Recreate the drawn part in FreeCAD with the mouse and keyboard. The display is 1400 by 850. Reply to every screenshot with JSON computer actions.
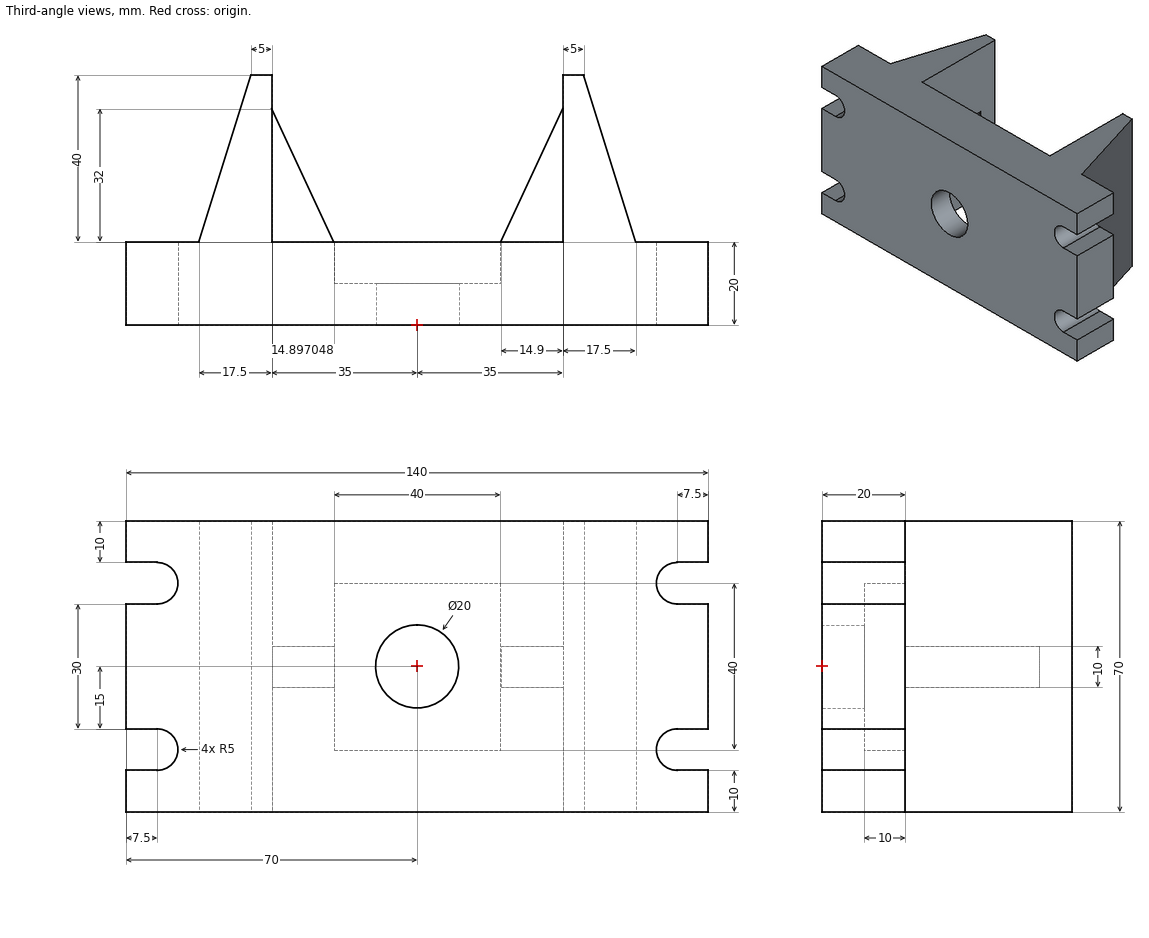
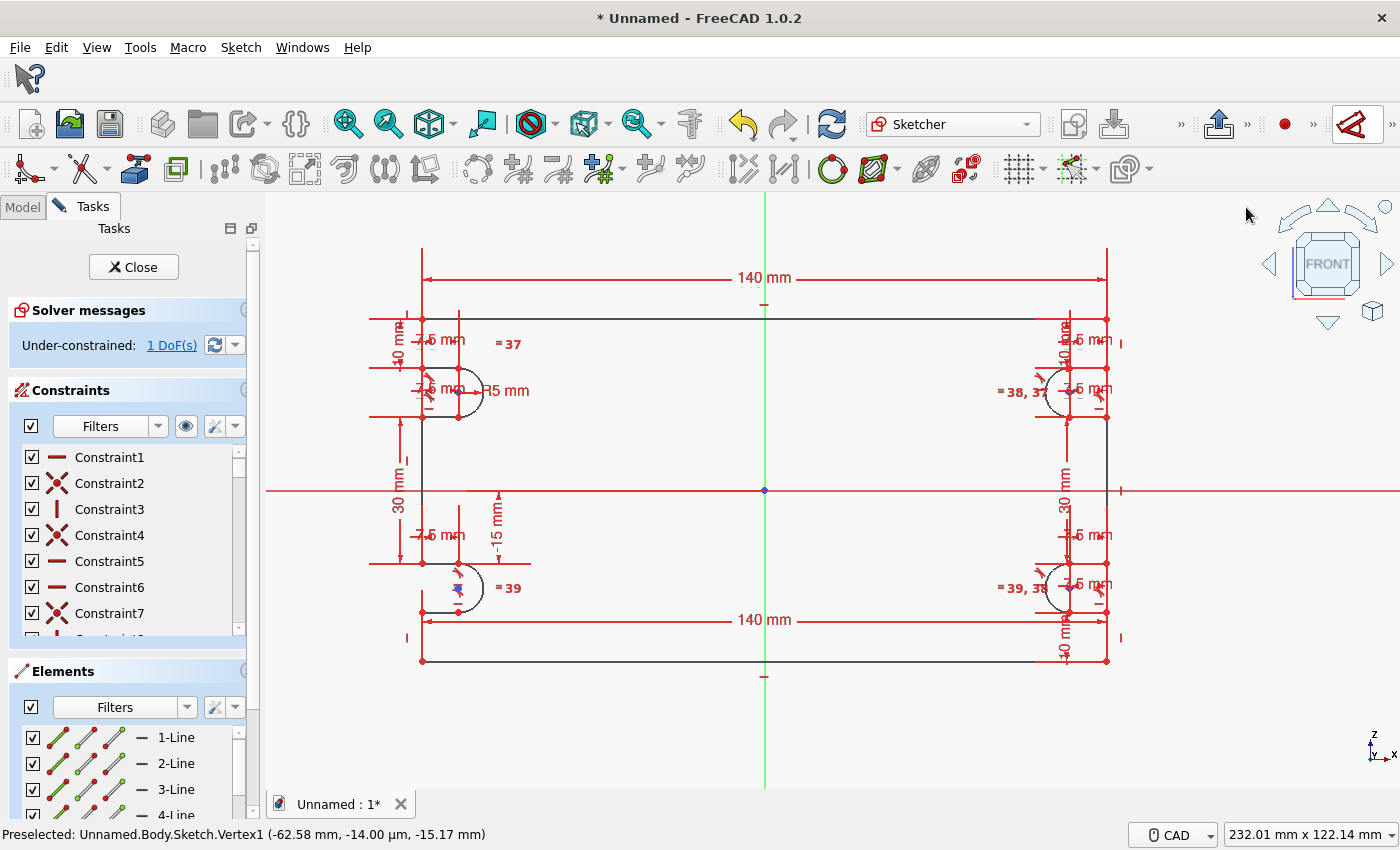
{"action": "left_click", "coordinate": [422, 564]}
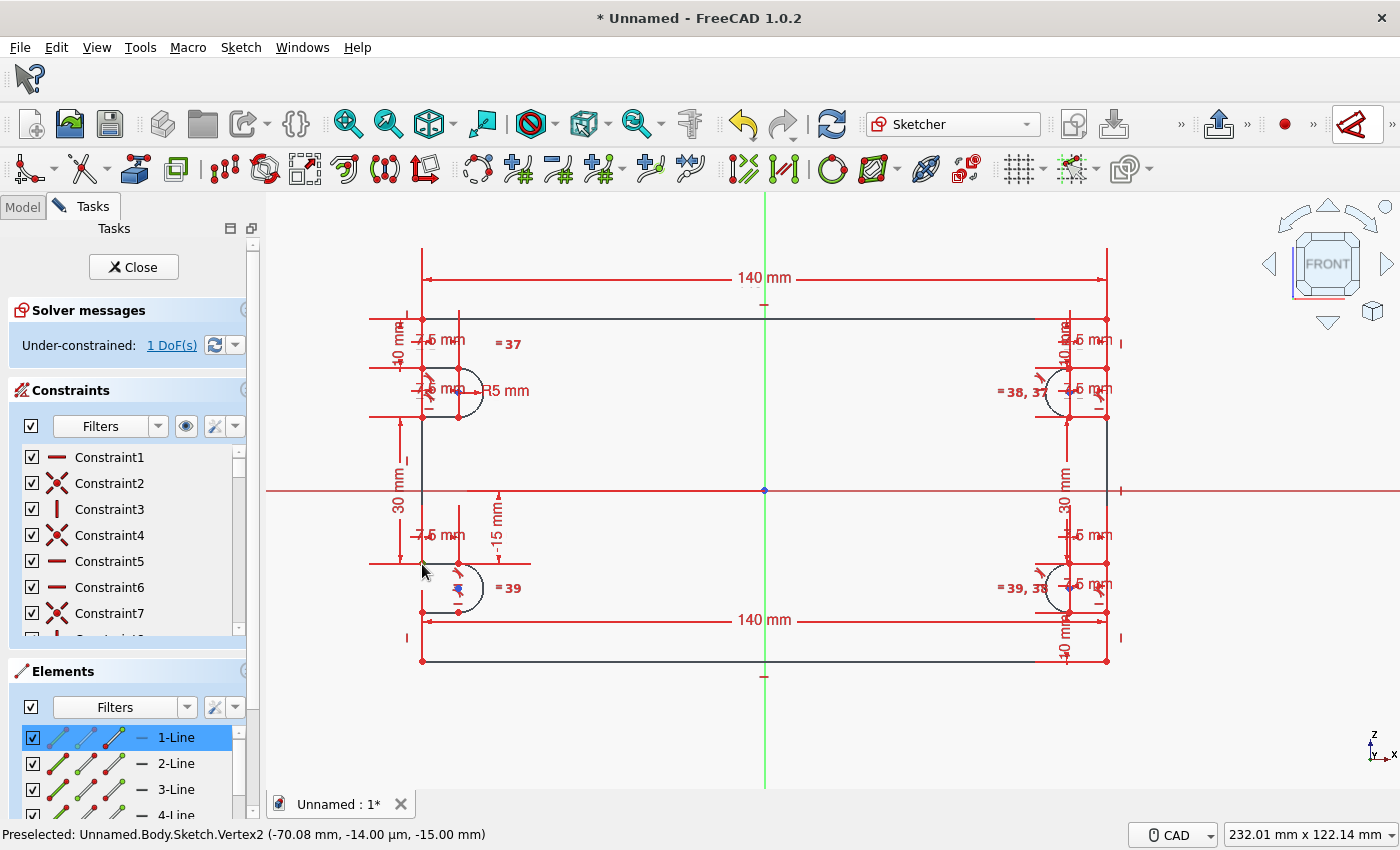
{"action": "left_click", "coordinate": [1378, 124]}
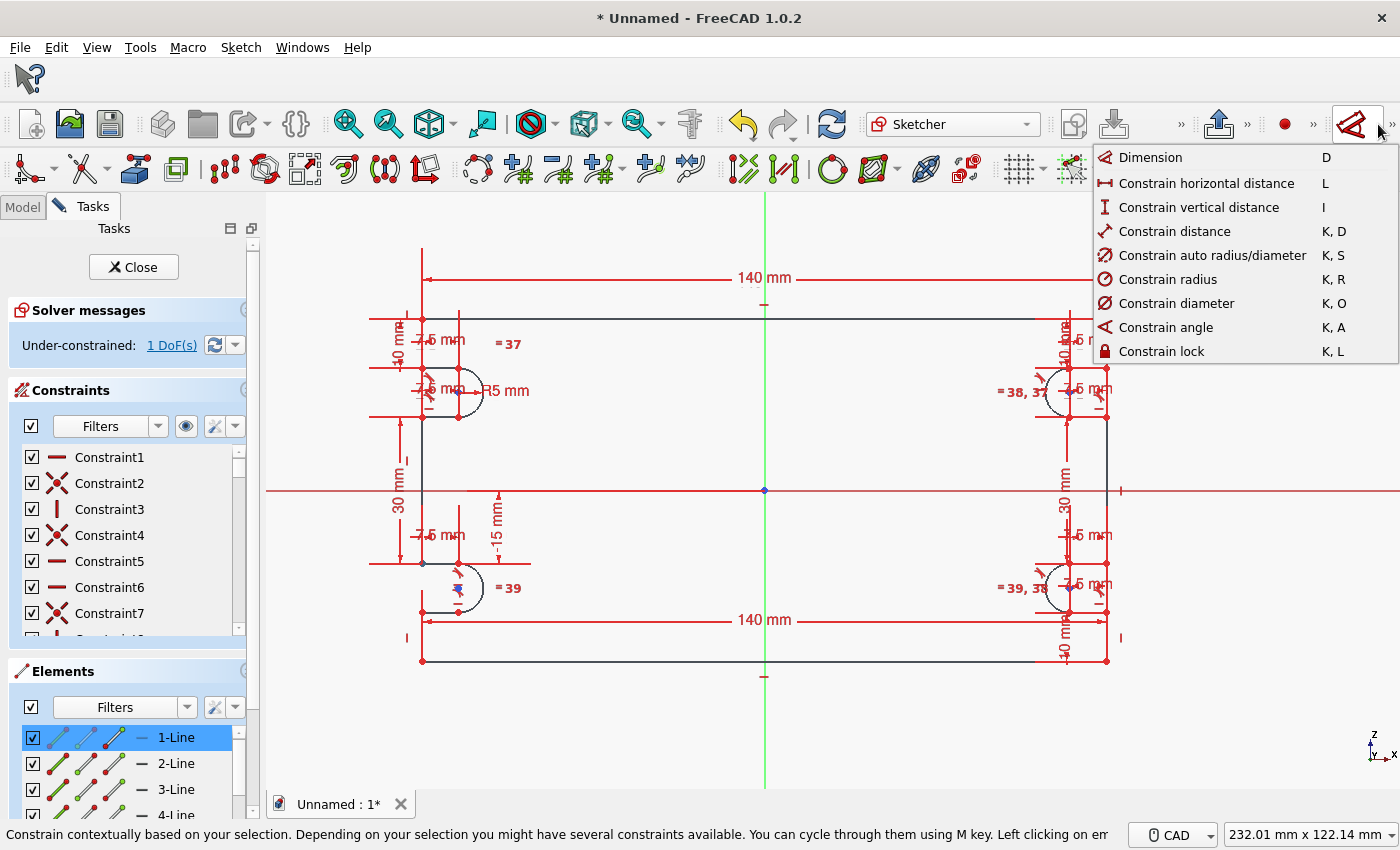
{"action": "left_click", "coordinate": [1246, 183]}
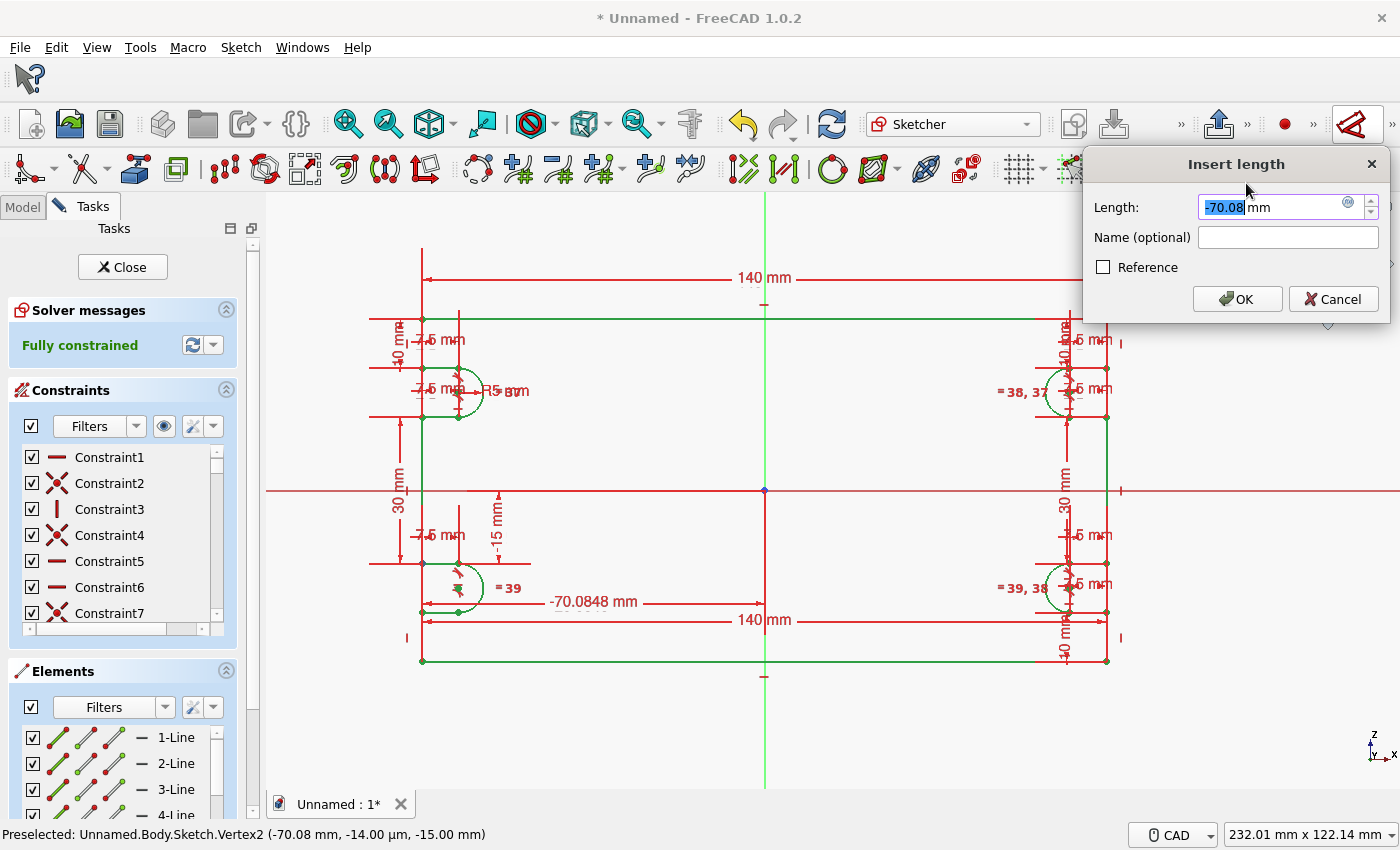
{"action": "type", "text": "-70"}
{"action": "key", "text": "Return"}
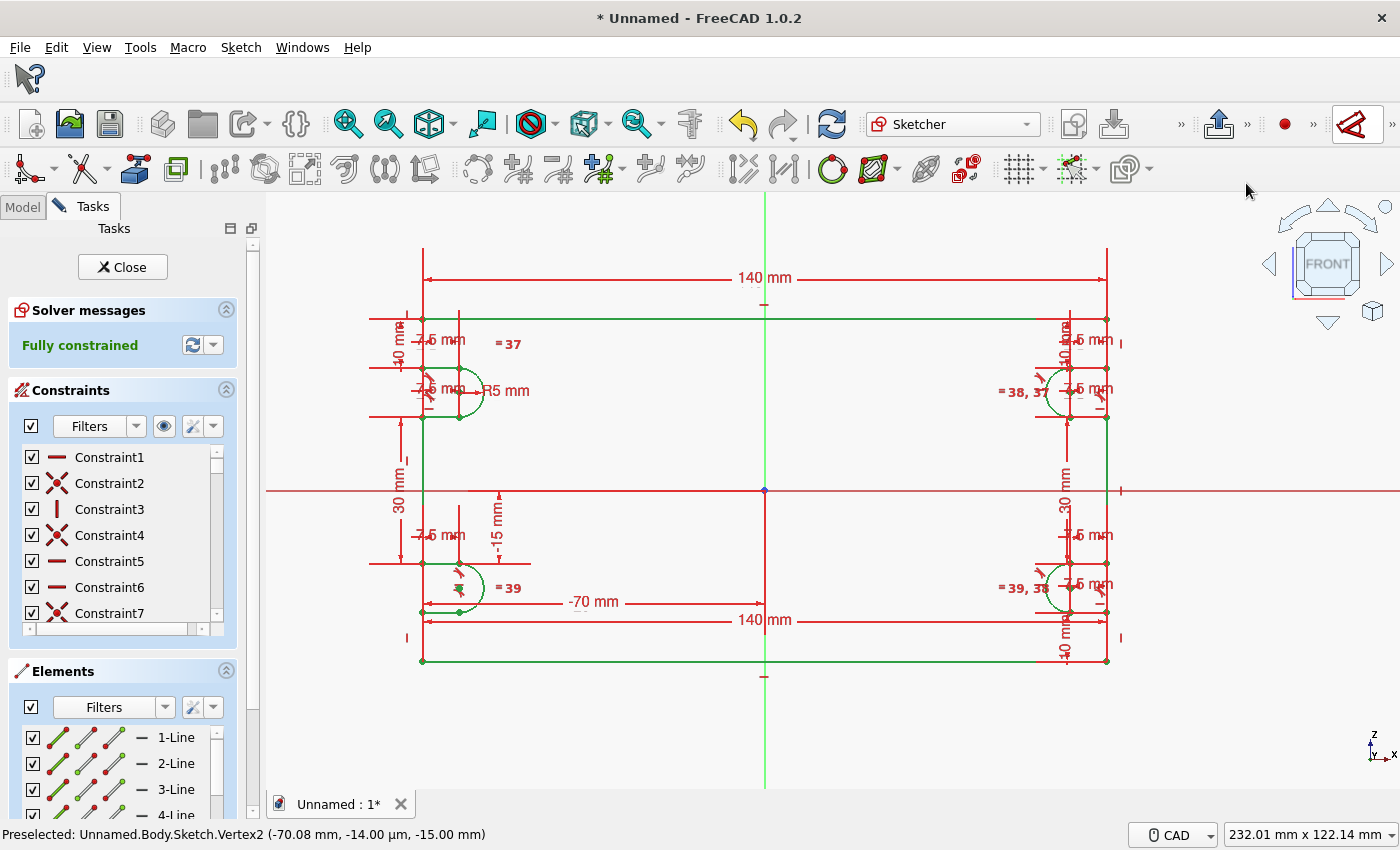
{"action": "left_click", "coordinate": [123, 267]}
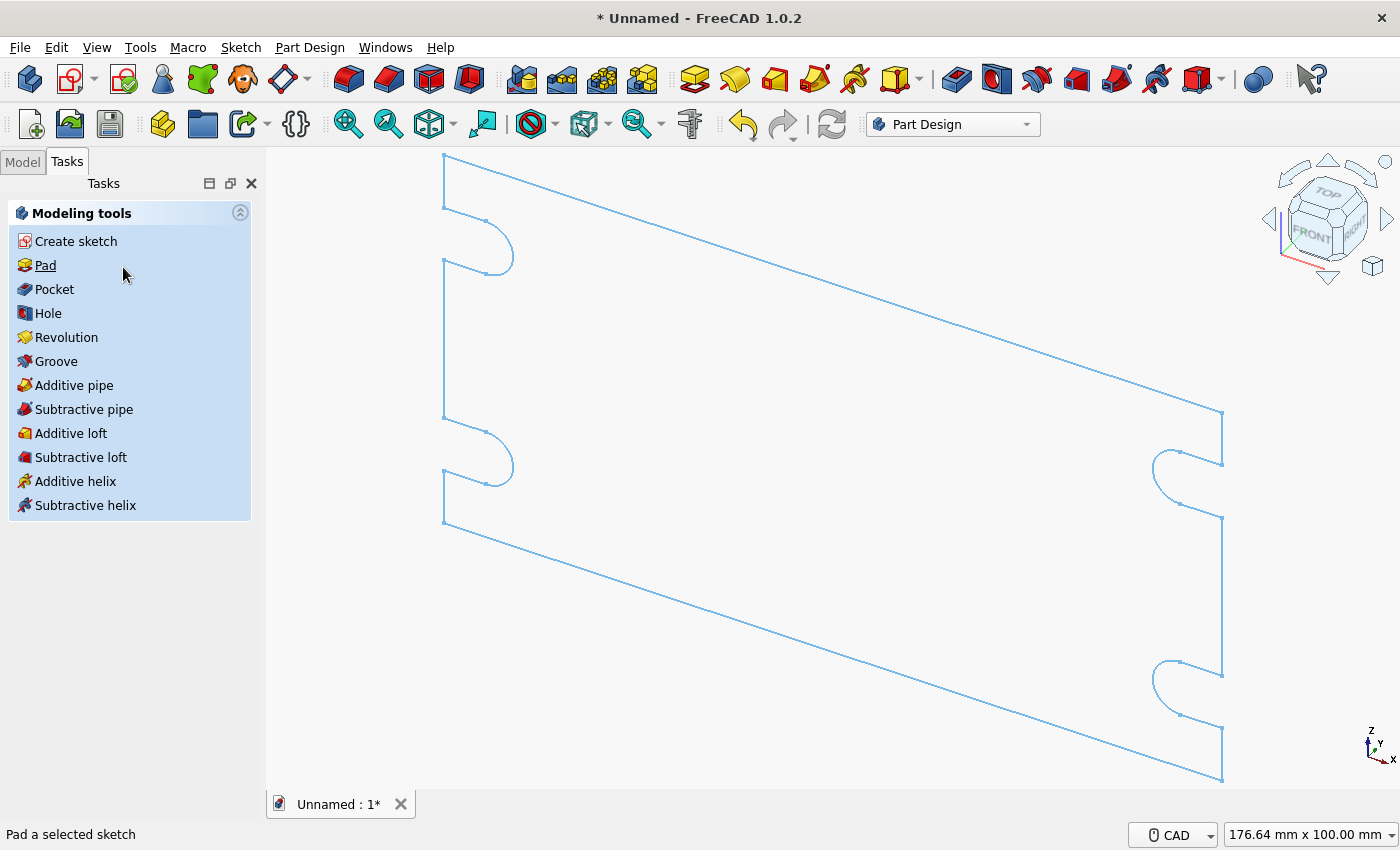
{"action": "left_click", "coordinate": [696, 80]}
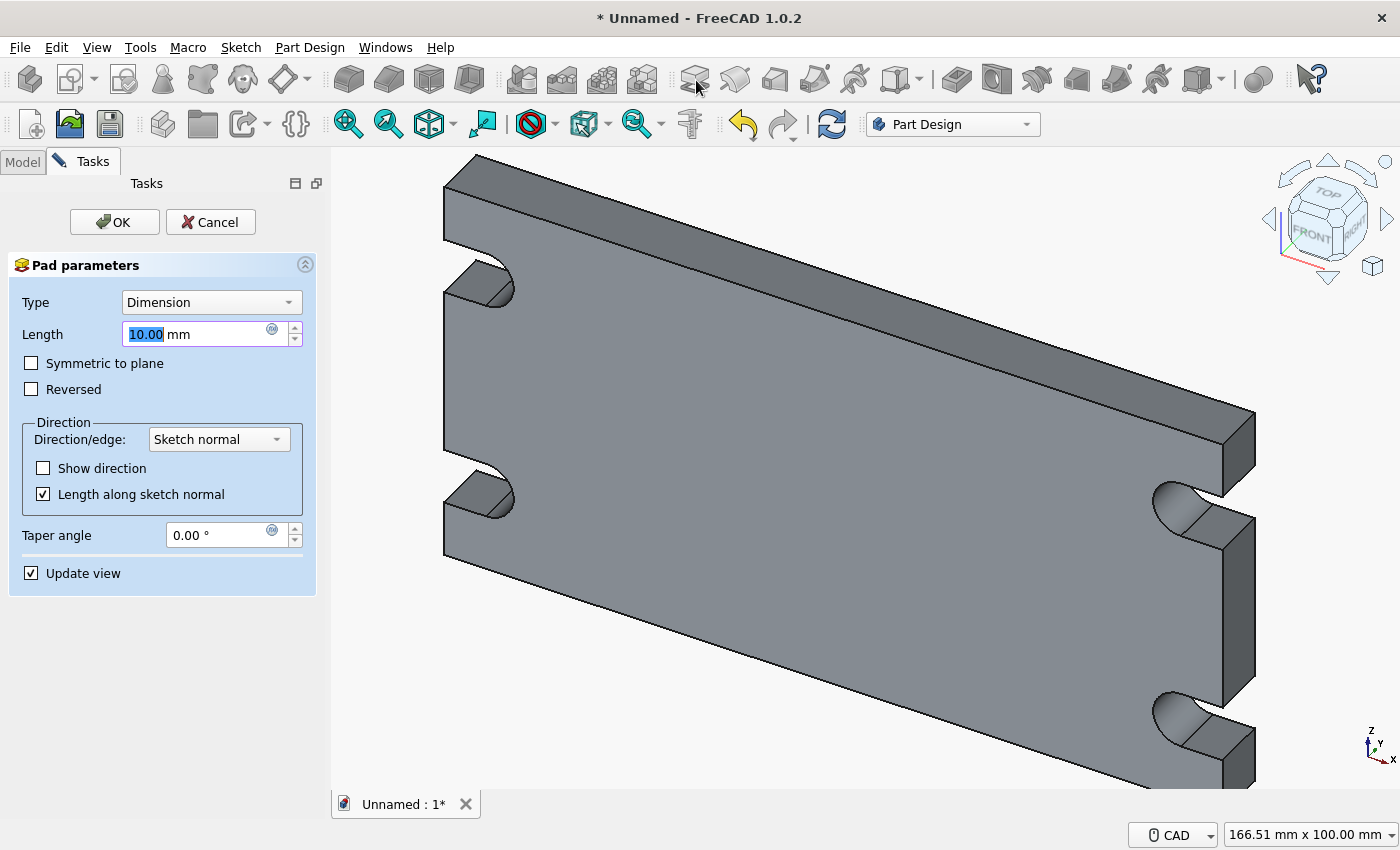
{"action": "type", "text": "20"}
{"action": "key", "text": "Tab"}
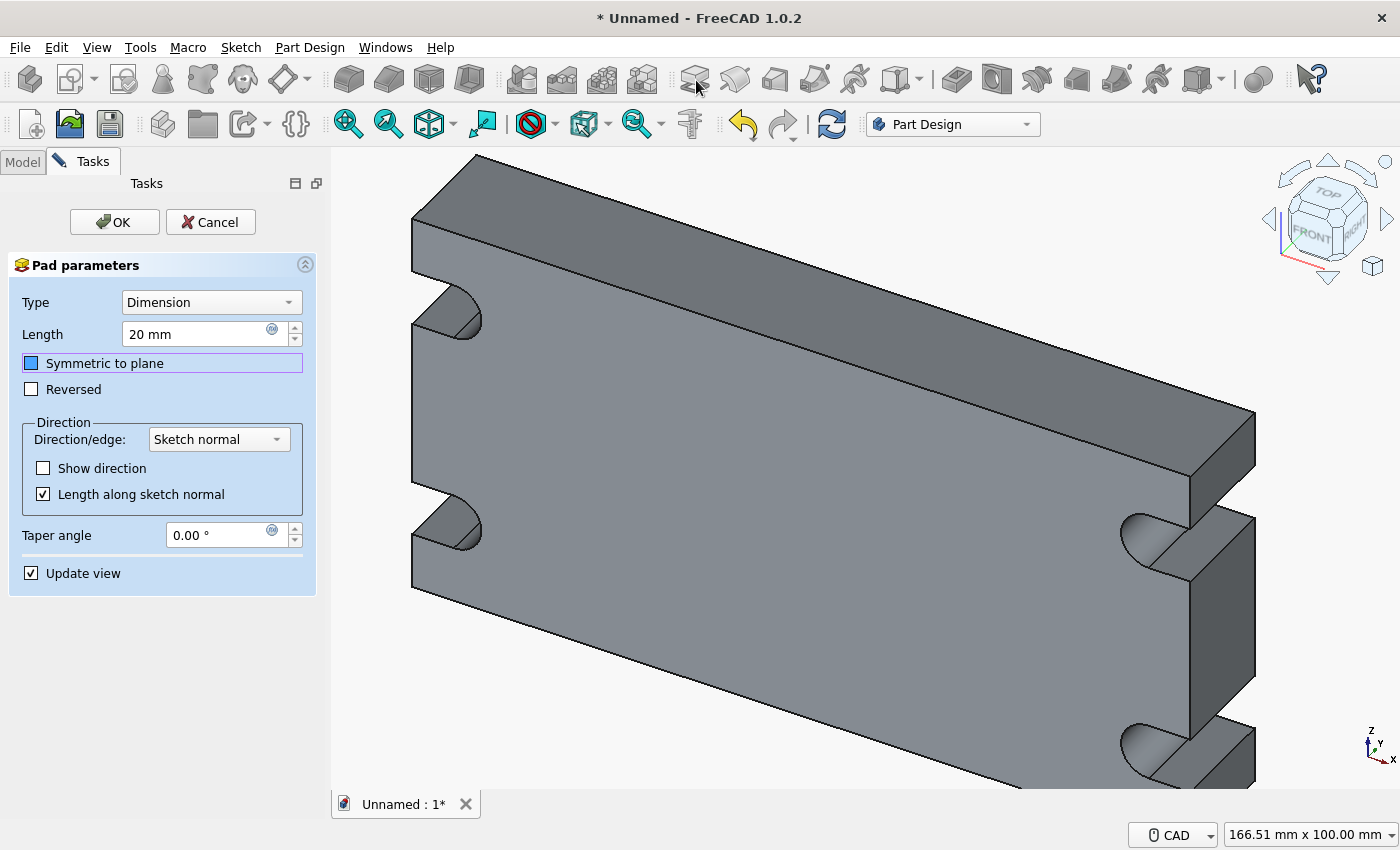
{"action": "left_click", "coordinate": [30, 389]}